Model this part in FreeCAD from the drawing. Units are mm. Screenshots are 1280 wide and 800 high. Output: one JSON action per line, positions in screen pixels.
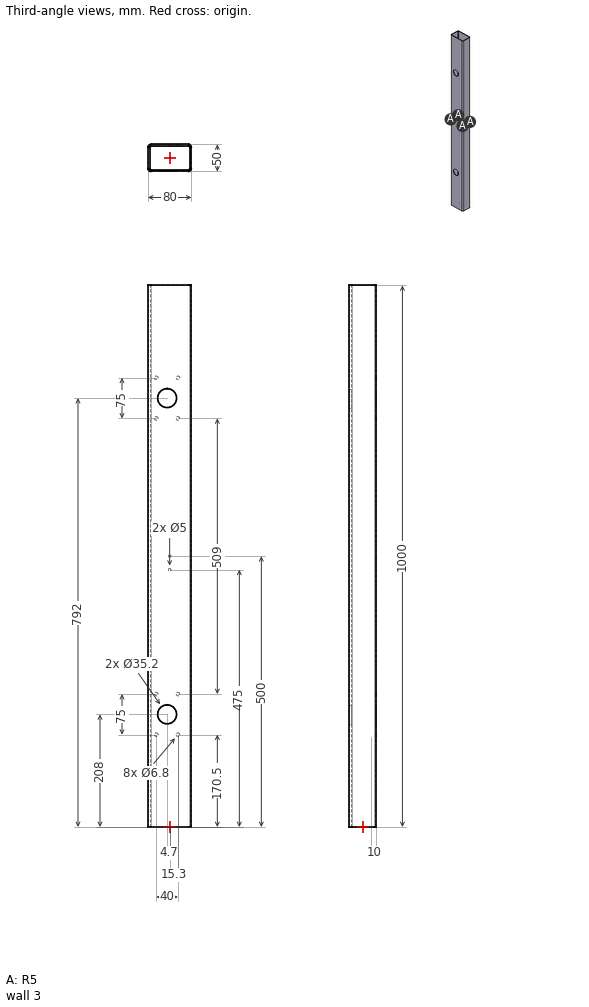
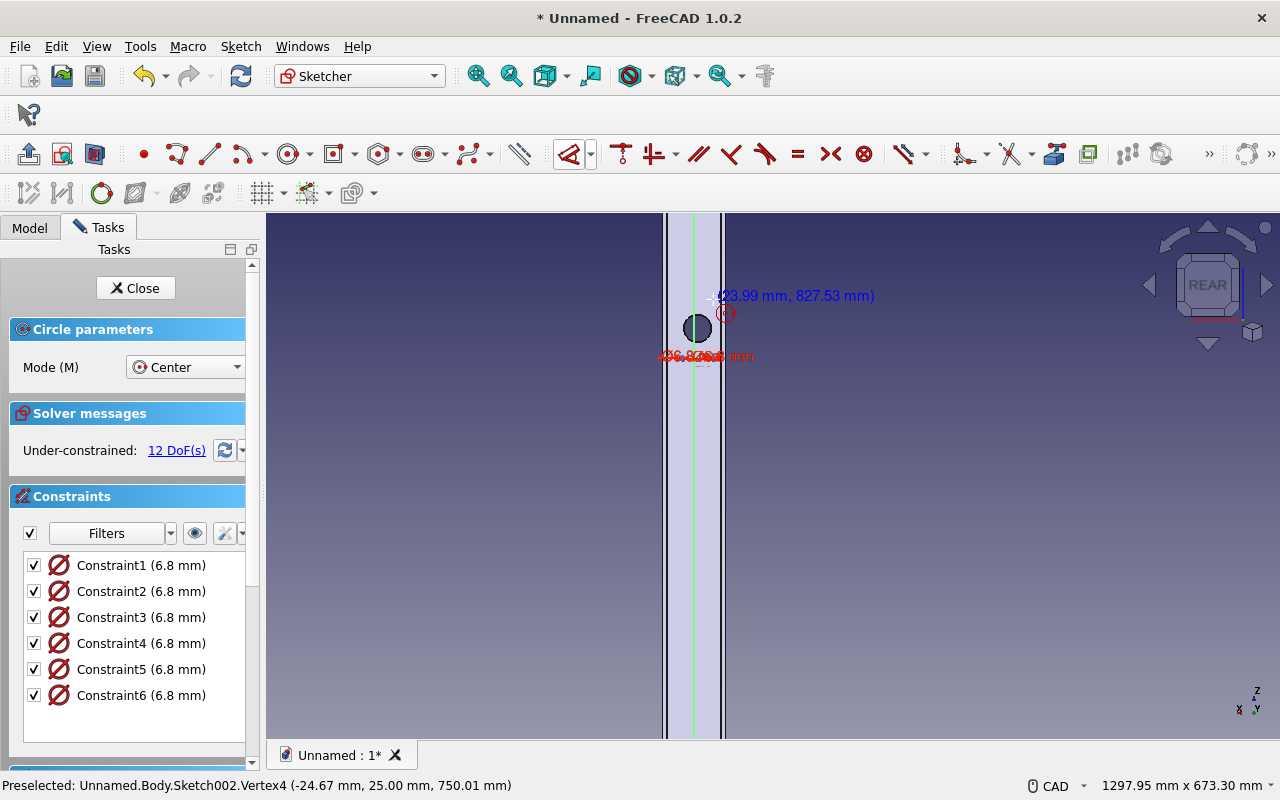
{"action": "left_click", "coordinate": [713, 299]}
{"action": "mouse_move", "coordinate": [715, 297]}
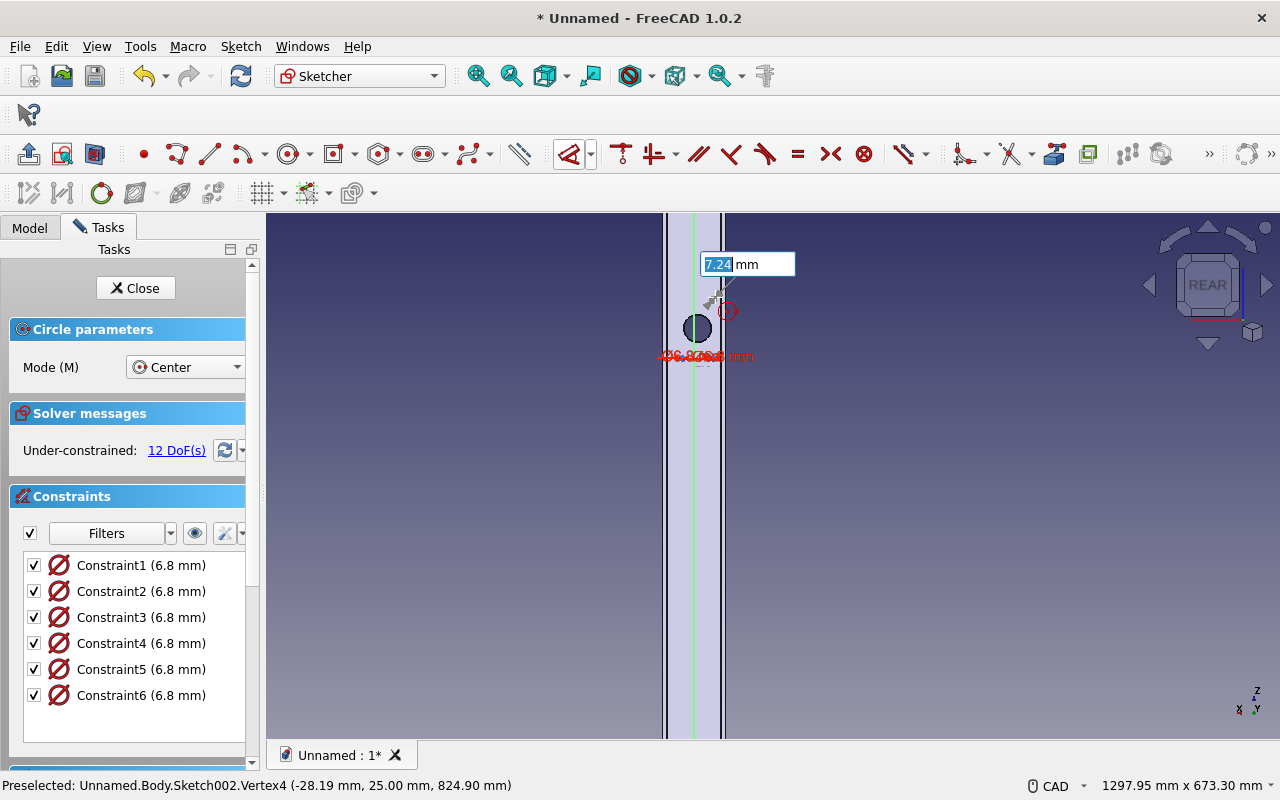
{"action": "type", "text": "6.8"}
{"action": "key", "text": "Return"}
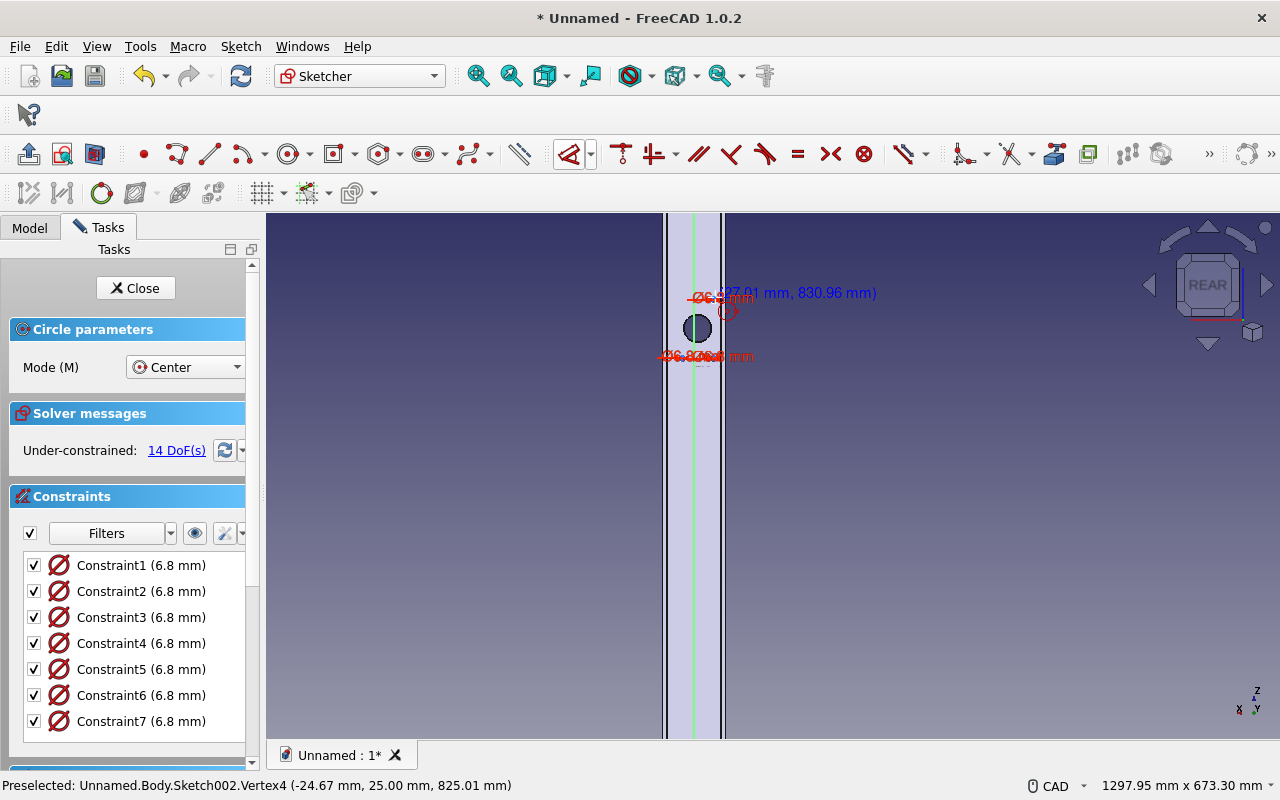
{"action": "scroll", "coordinate": [682, 299], "scroll_direction": "up", "scroll_amount": 11}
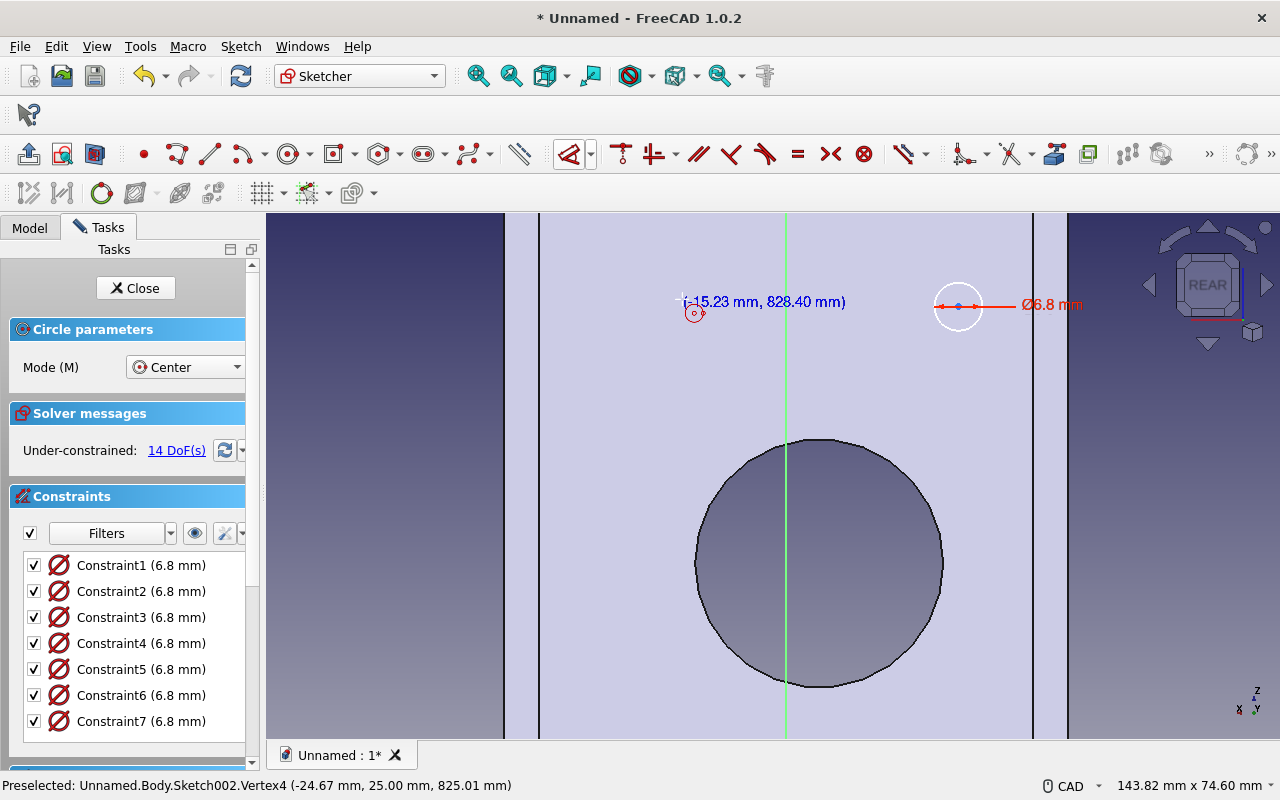
{"action": "scroll", "coordinate": [697, 299], "scroll_direction": "down", "scroll_amount": 14}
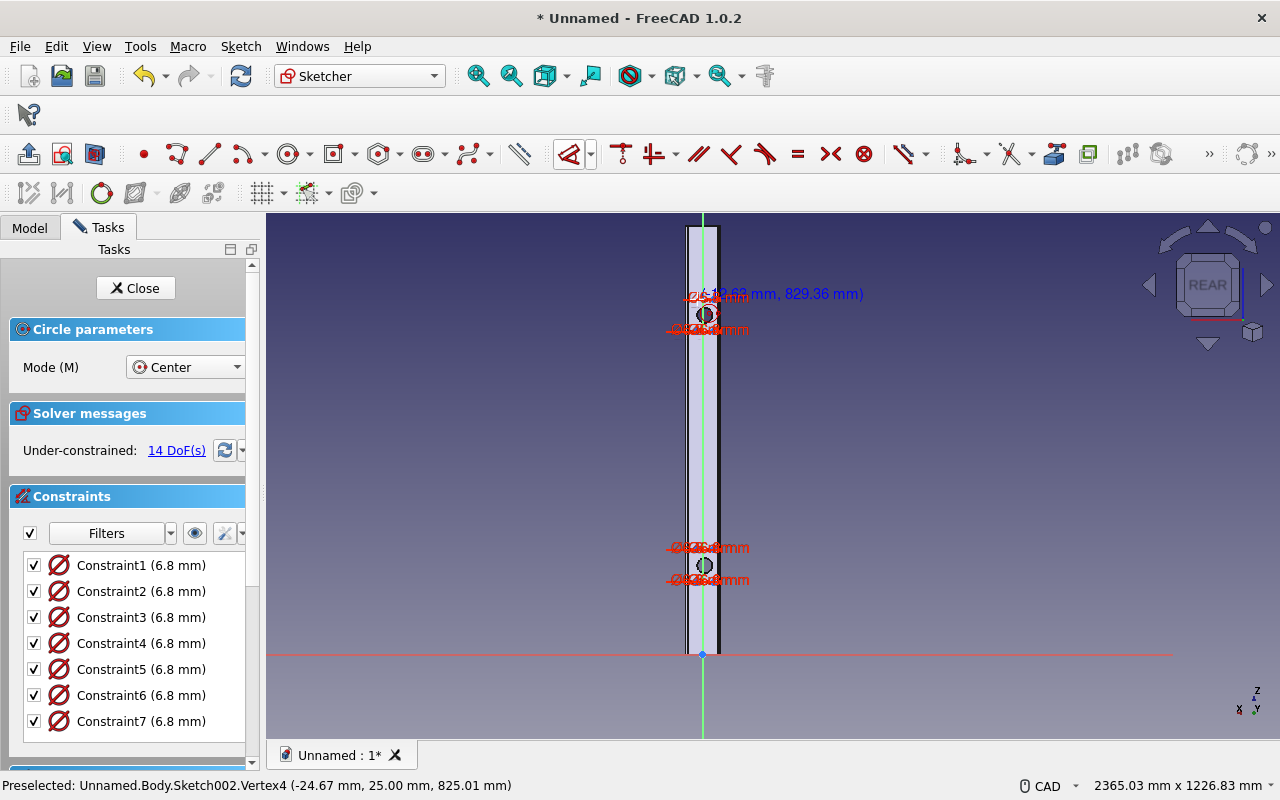
{"action": "scroll", "coordinate": [696, 299], "scroll_direction": "up", "scroll_amount": 5}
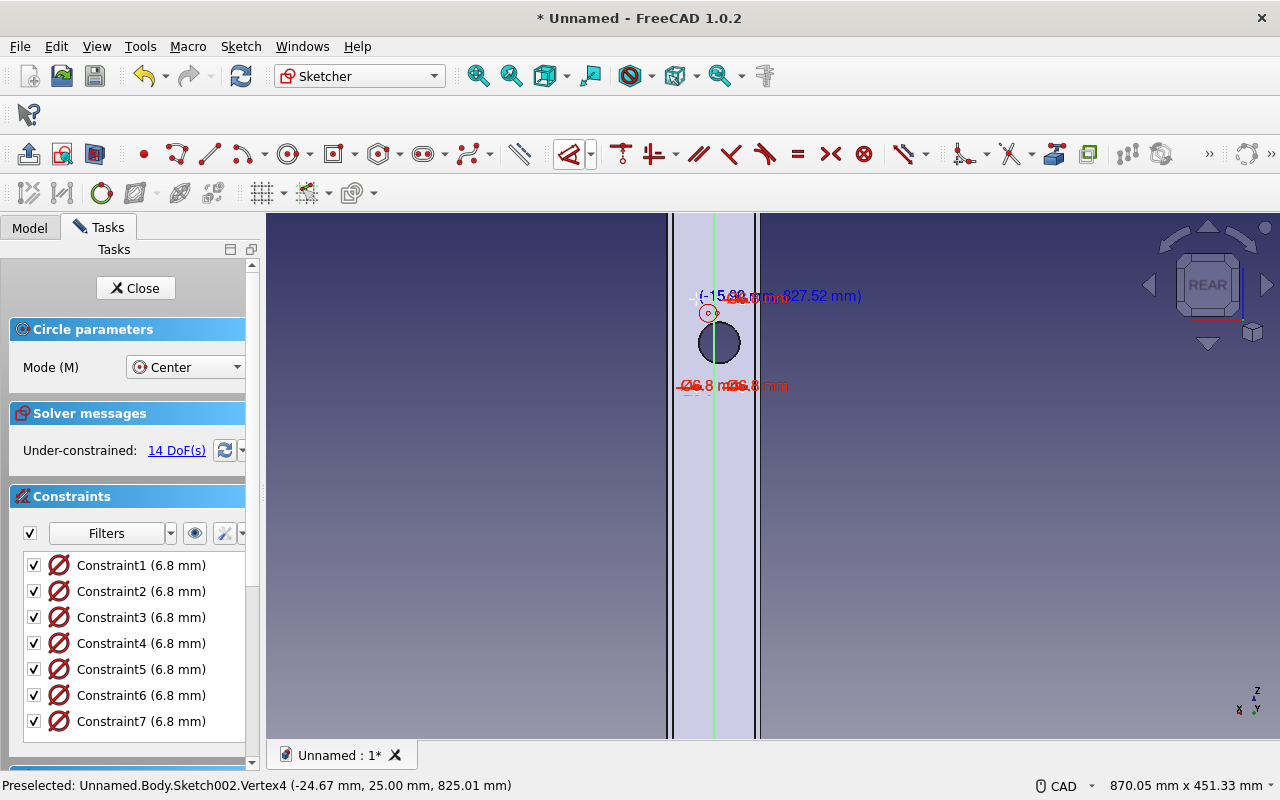
{"action": "left_click", "coordinate": [696, 299]}
{"action": "mouse_move", "coordinate": [699, 296]}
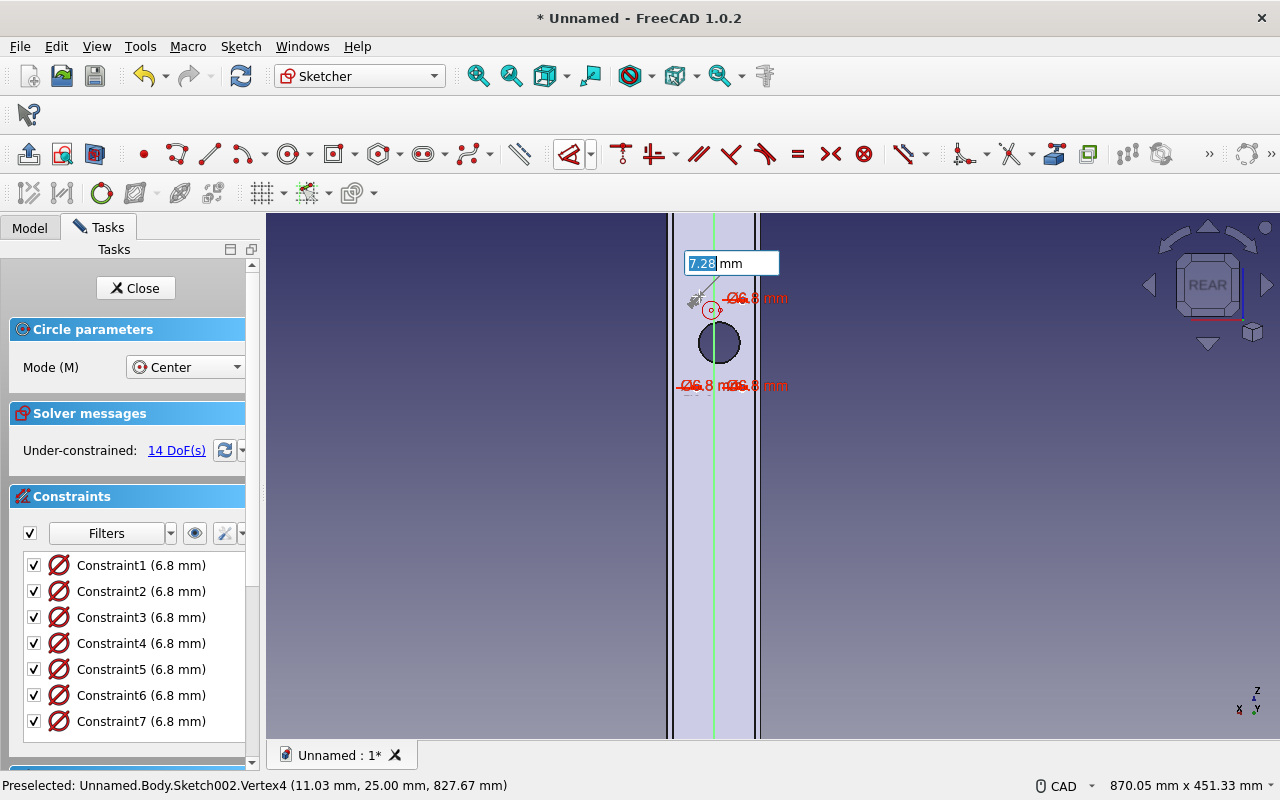
{"action": "type", "text": "6.8"}
{"action": "key", "text": "Return"}
{"action": "key", "text": "Escape"}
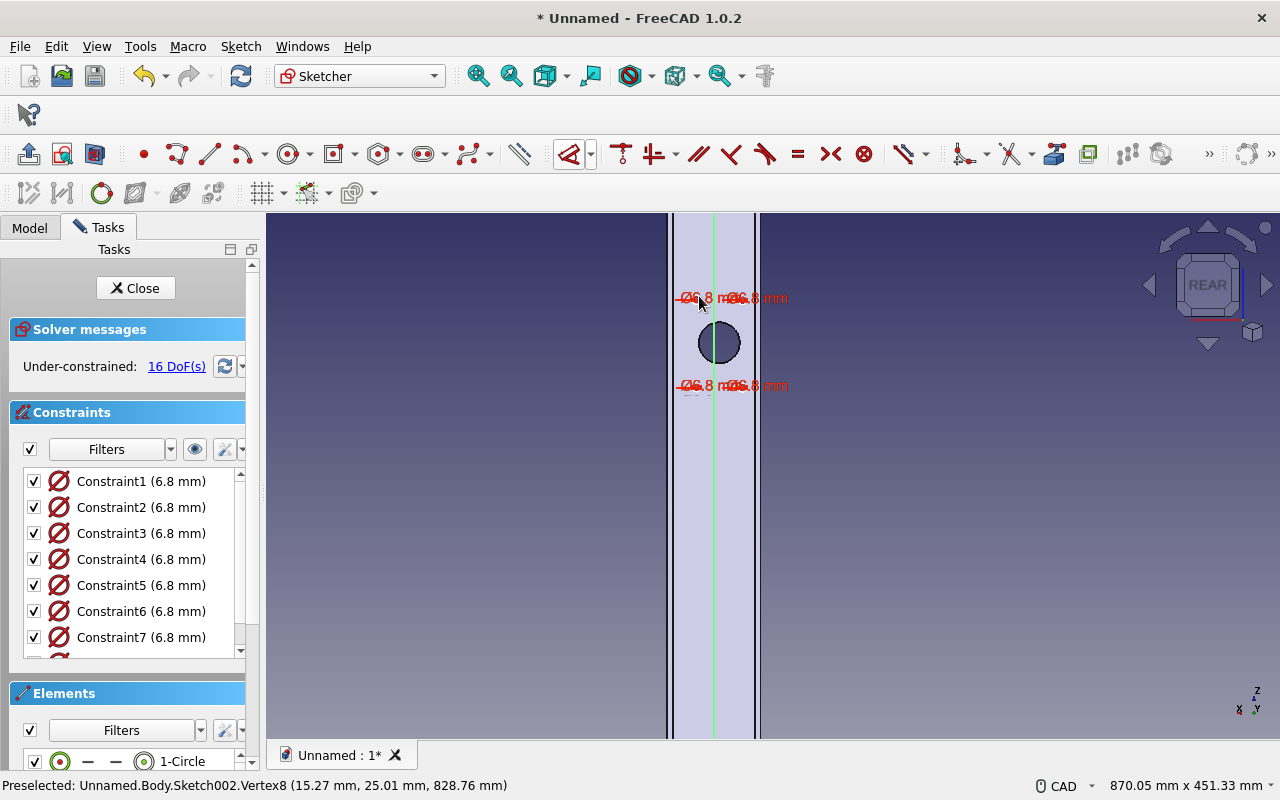
{"action": "scroll", "coordinate": [696, 299], "scroll_direction": "down", "scroll_amount": 5}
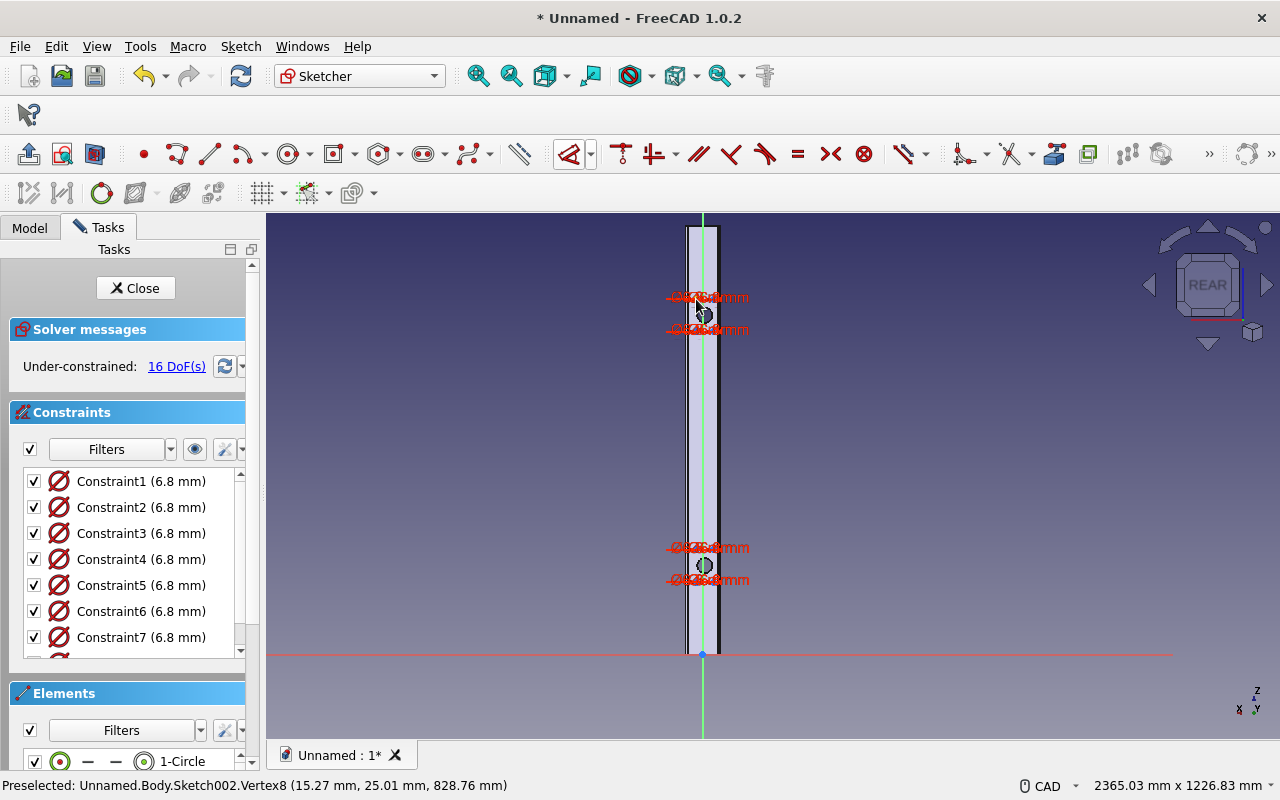
{"action": "scroll", "coordinate": [696, 582], "scroll_direction": "up", "scroll_amount": 5}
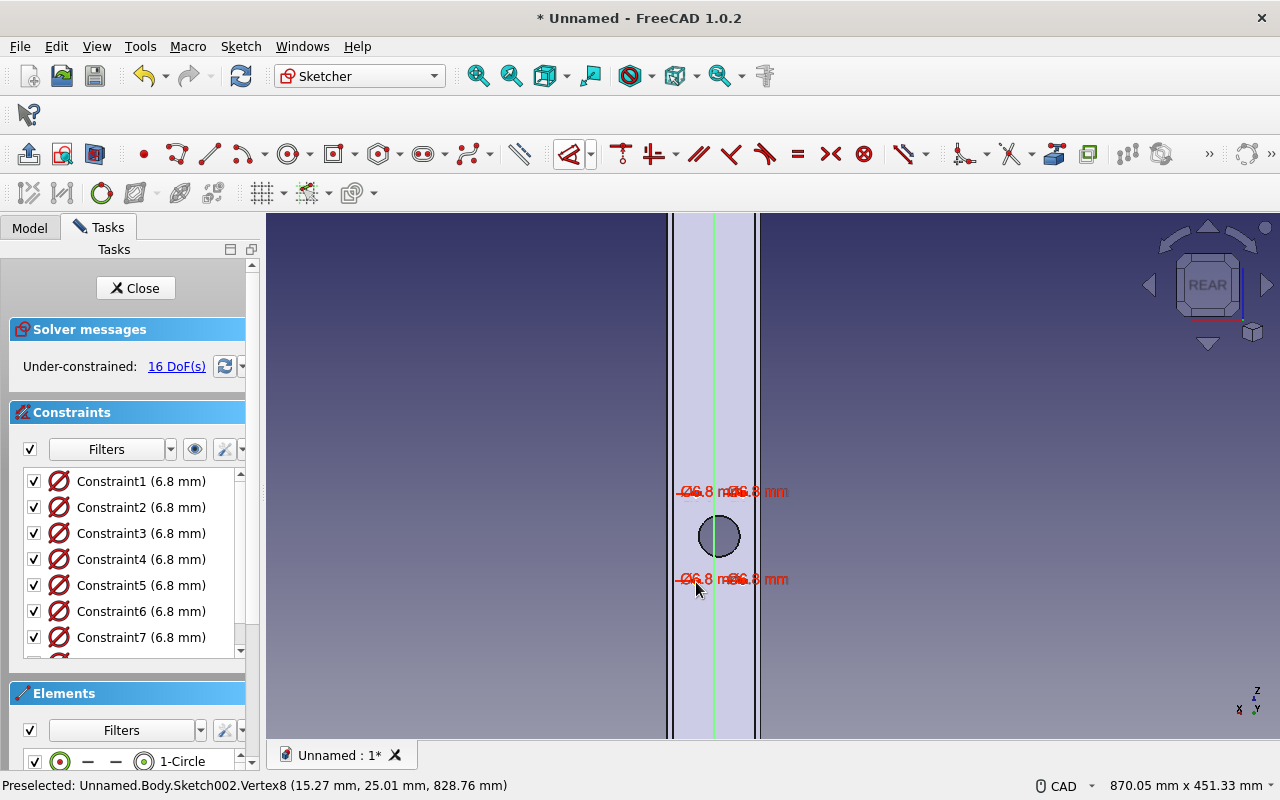
{"action": "left_click", "coordinate": [696, 581]}